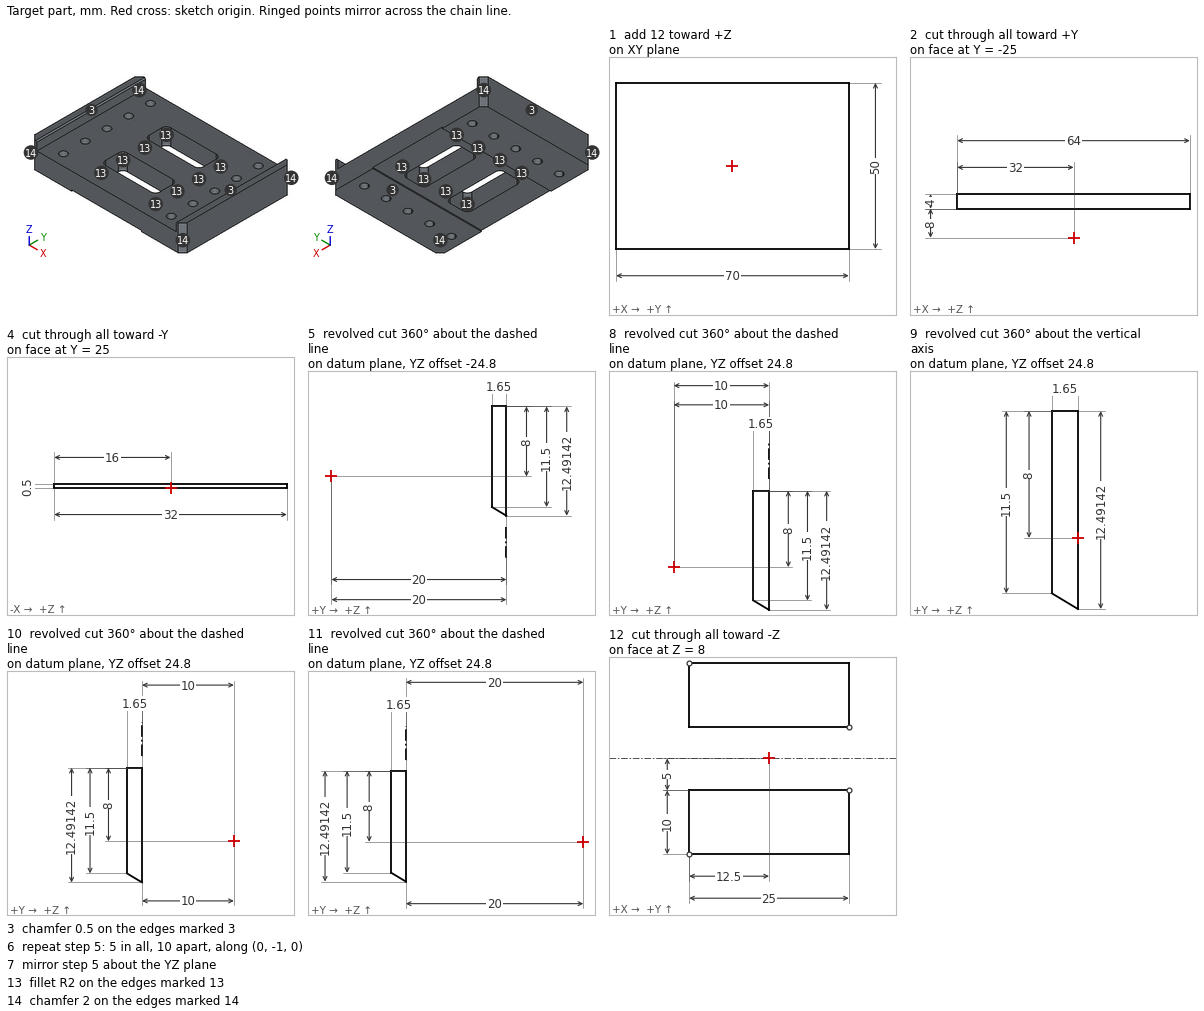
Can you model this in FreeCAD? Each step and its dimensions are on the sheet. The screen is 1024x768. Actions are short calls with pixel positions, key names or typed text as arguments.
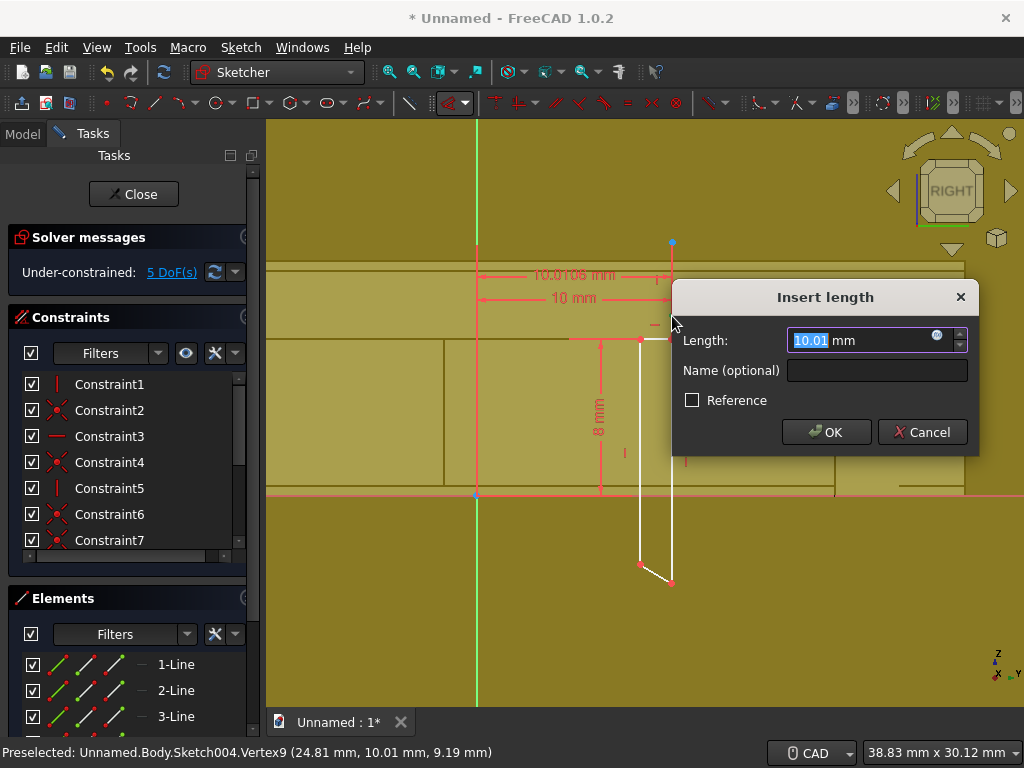
text(10)
key(Return)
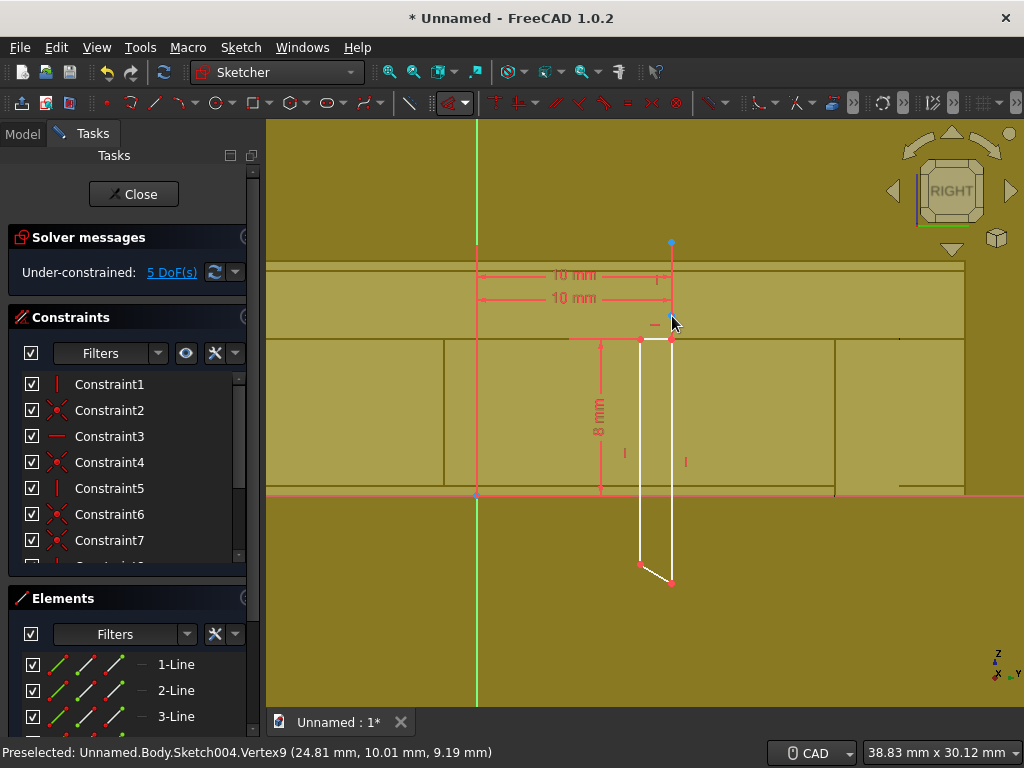
click(640, 497)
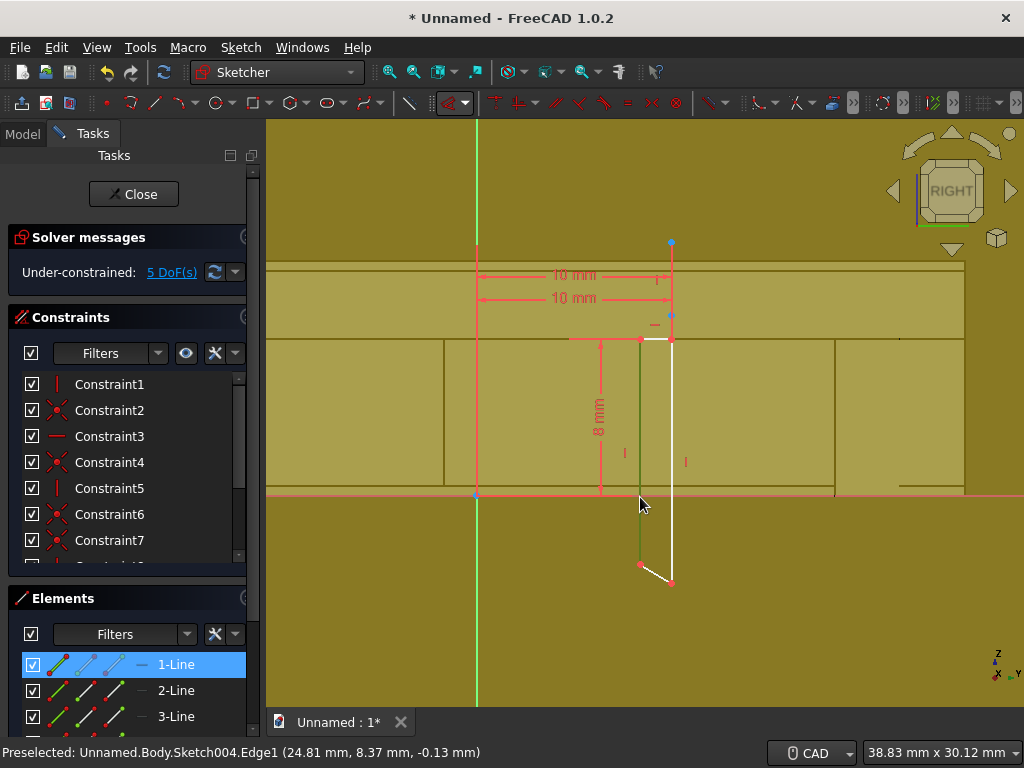
key(i)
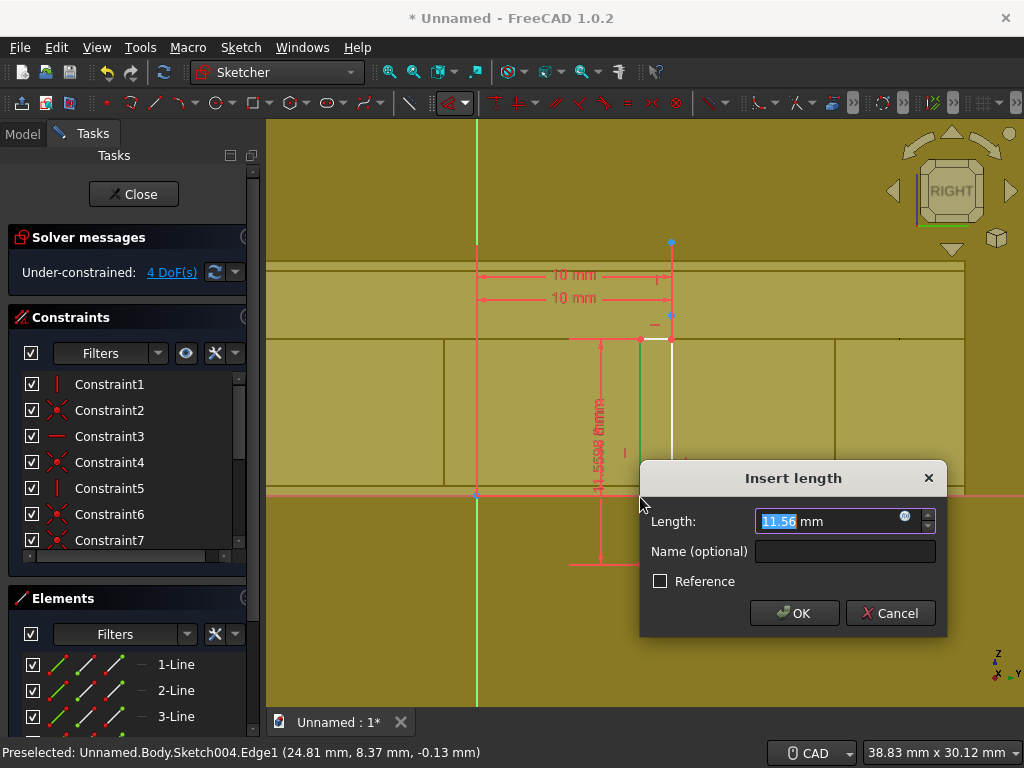
text(11.5)
key(Return)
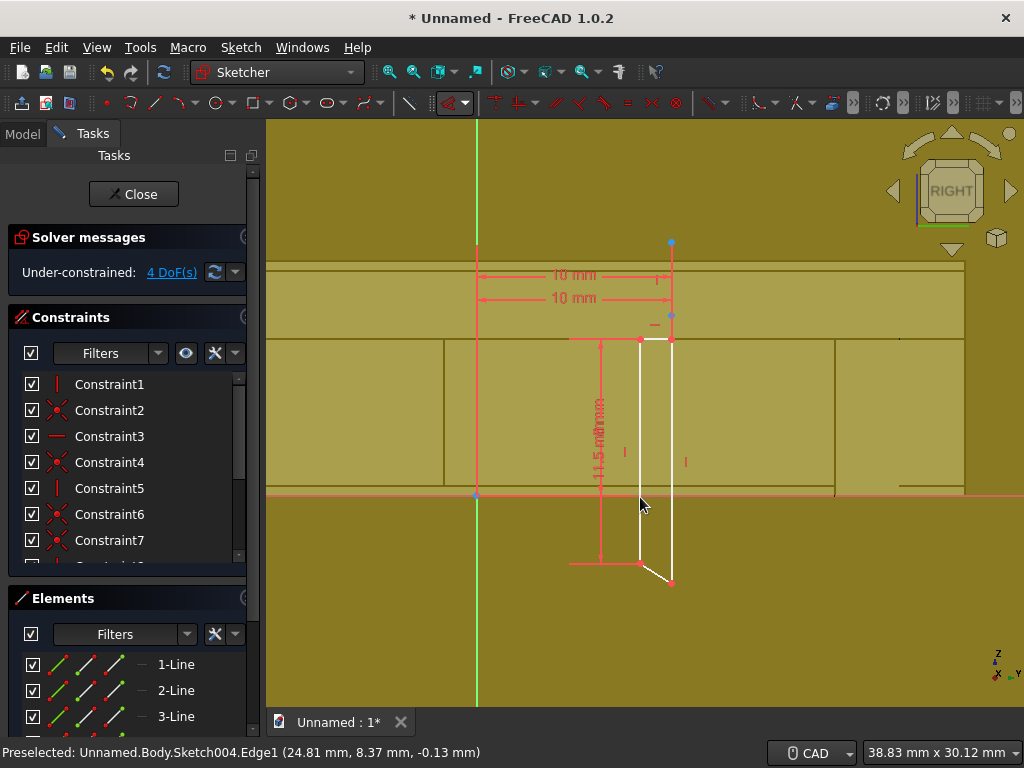
scroll(650, 339, up, 2)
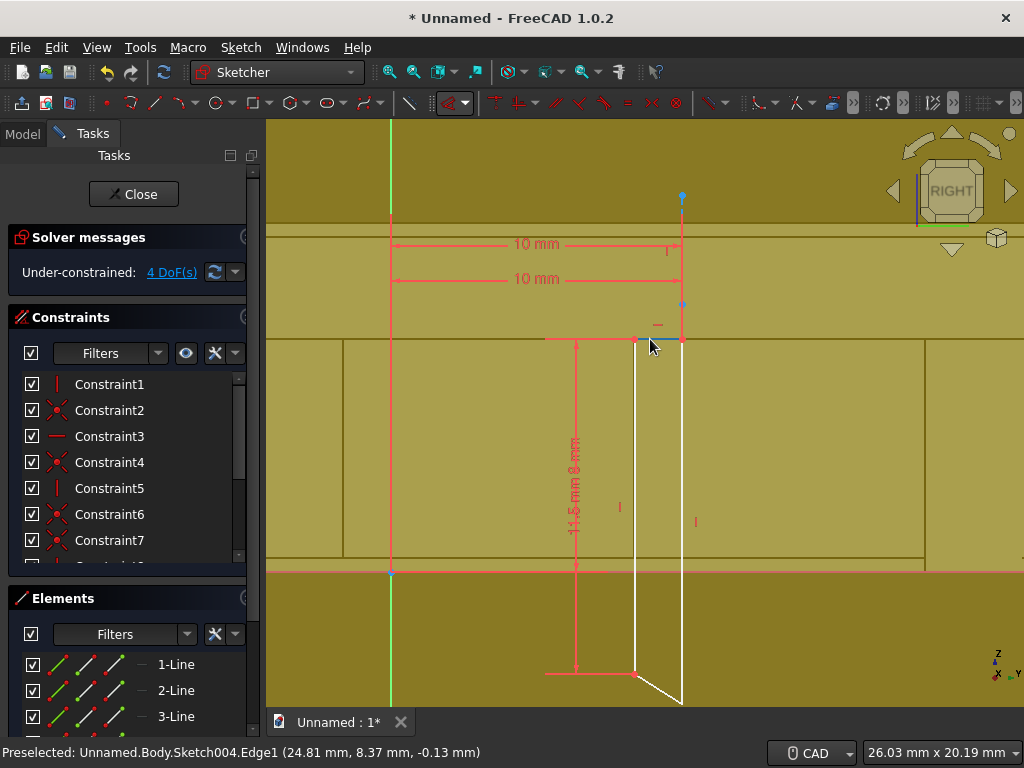
click(649, 339)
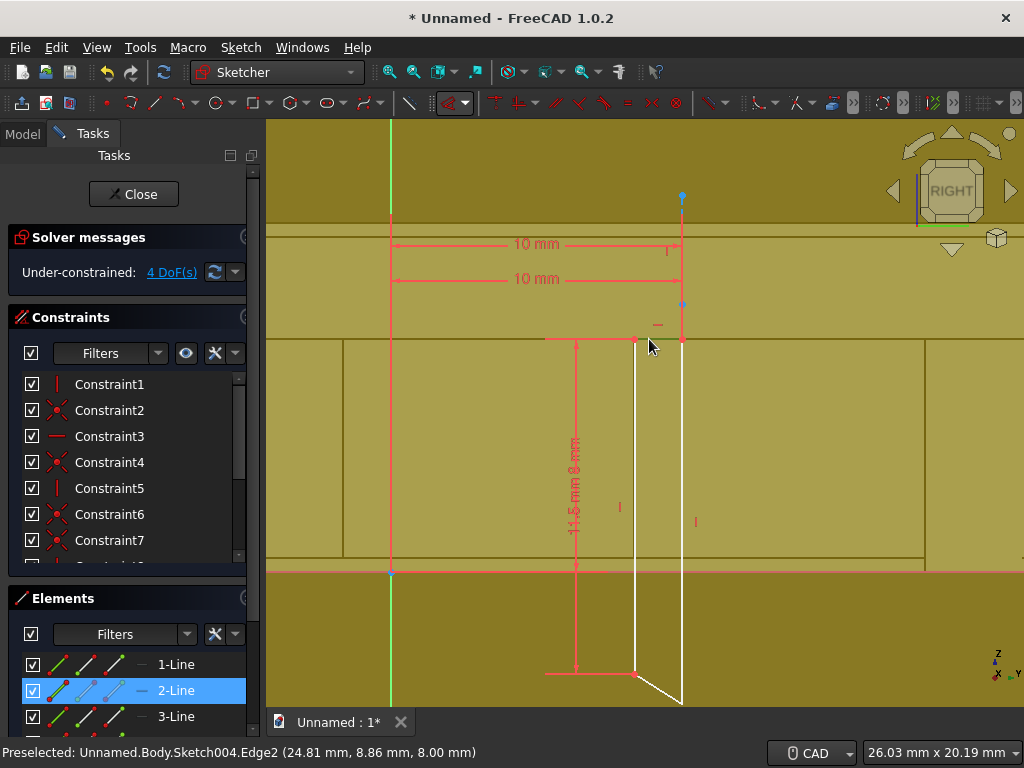
key(l)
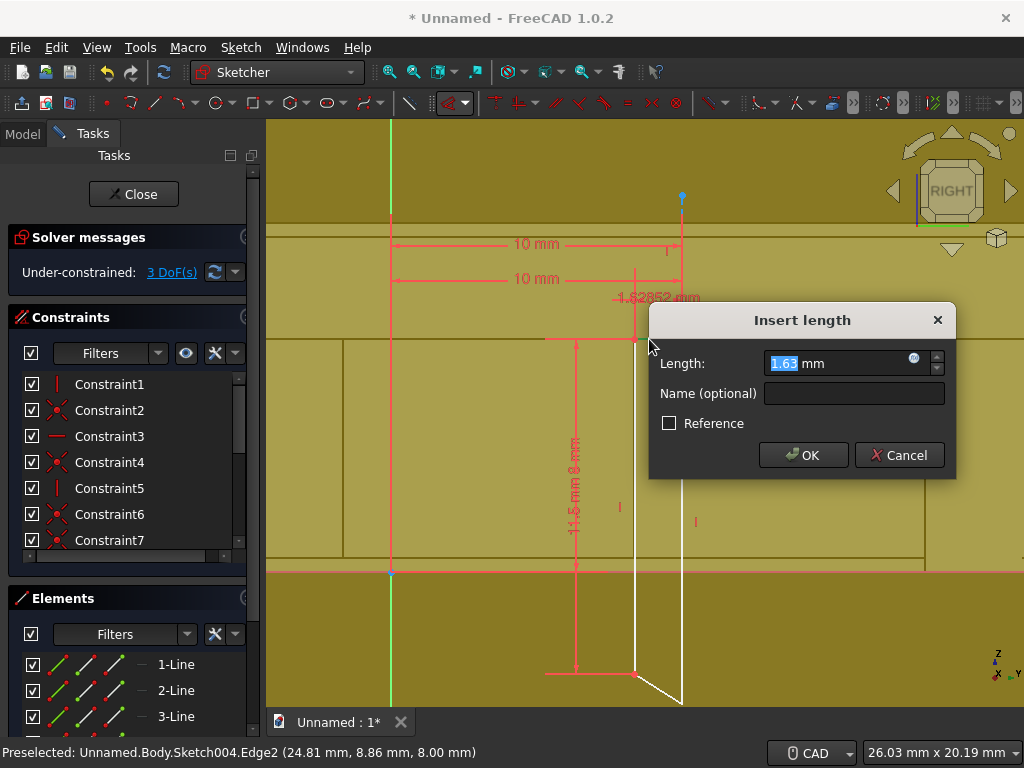
text(1.65)
key(Return)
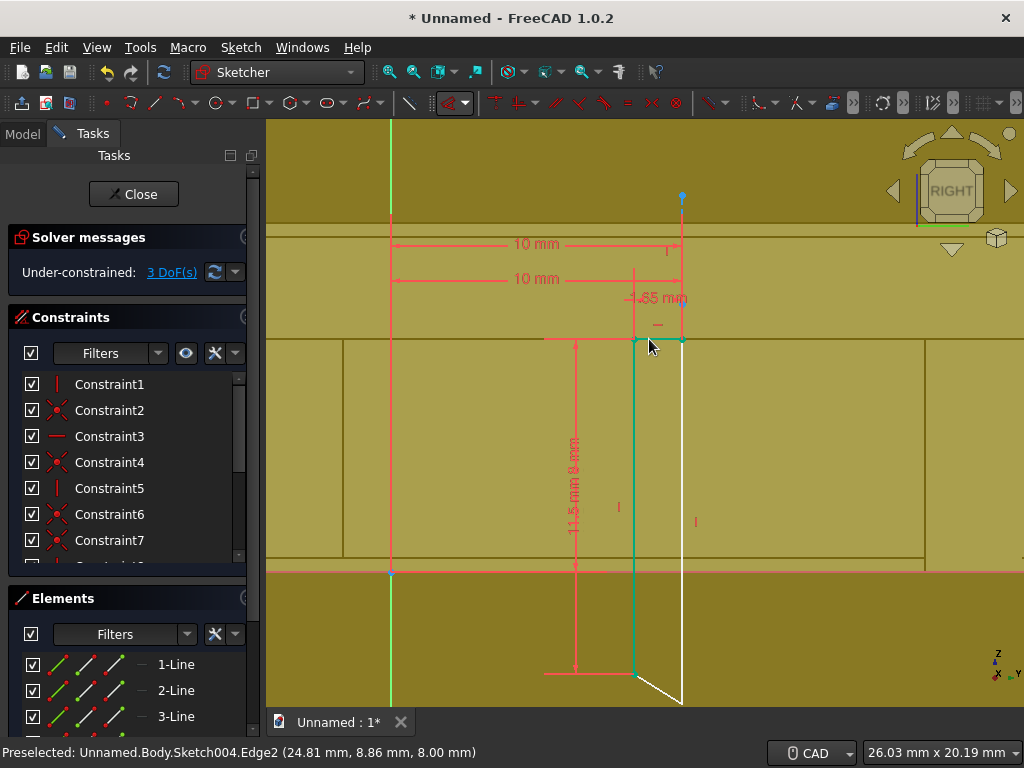
click(682, 449)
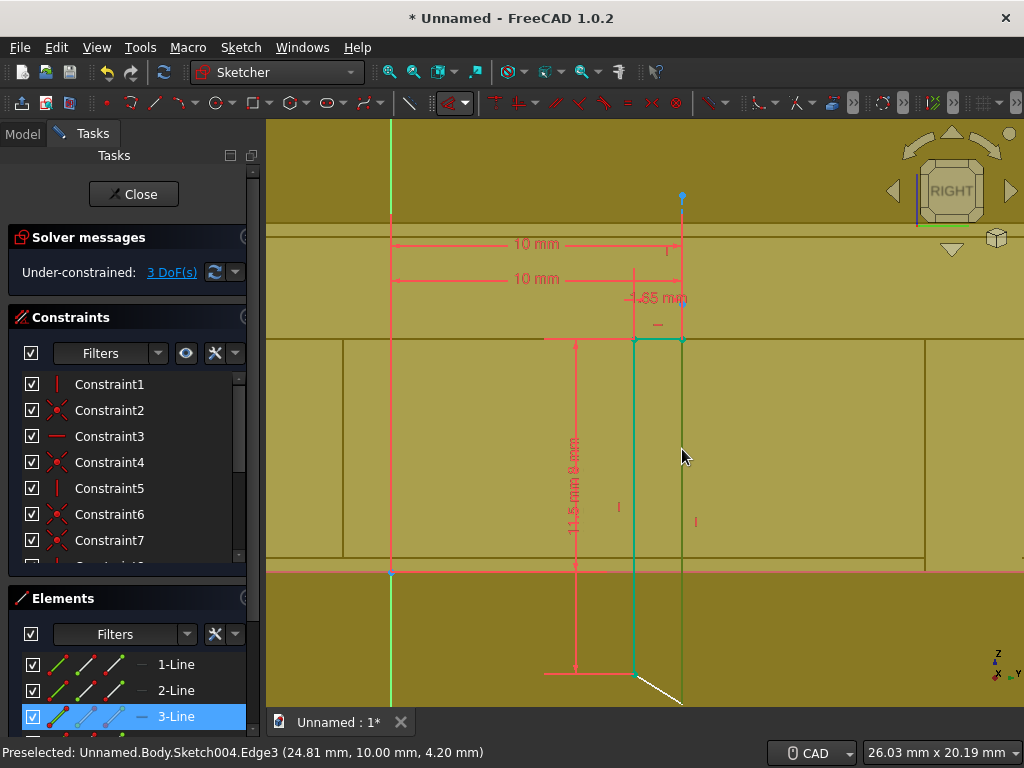
key(i)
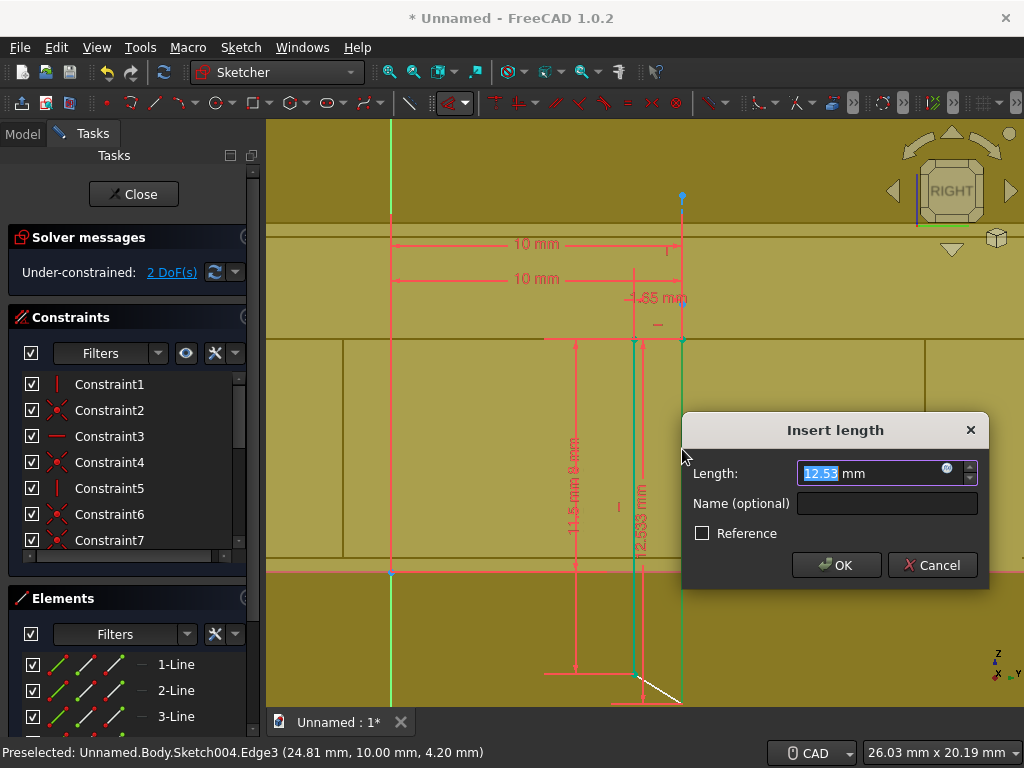
text(12.49142)
key(Return)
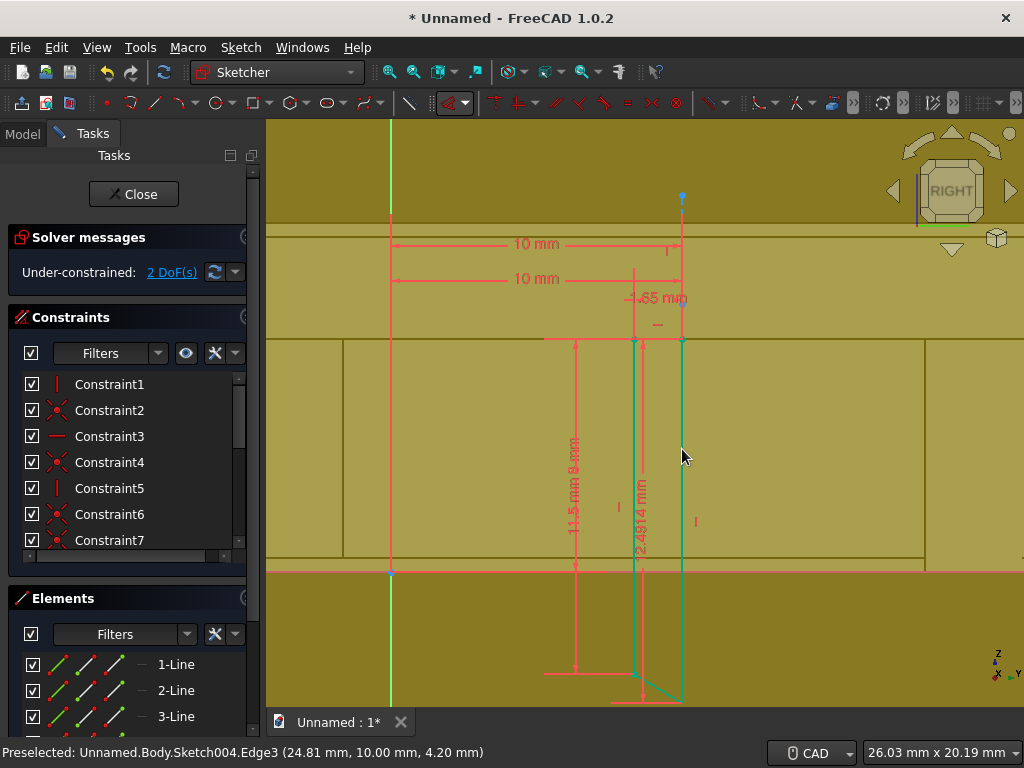
click(134, 194)